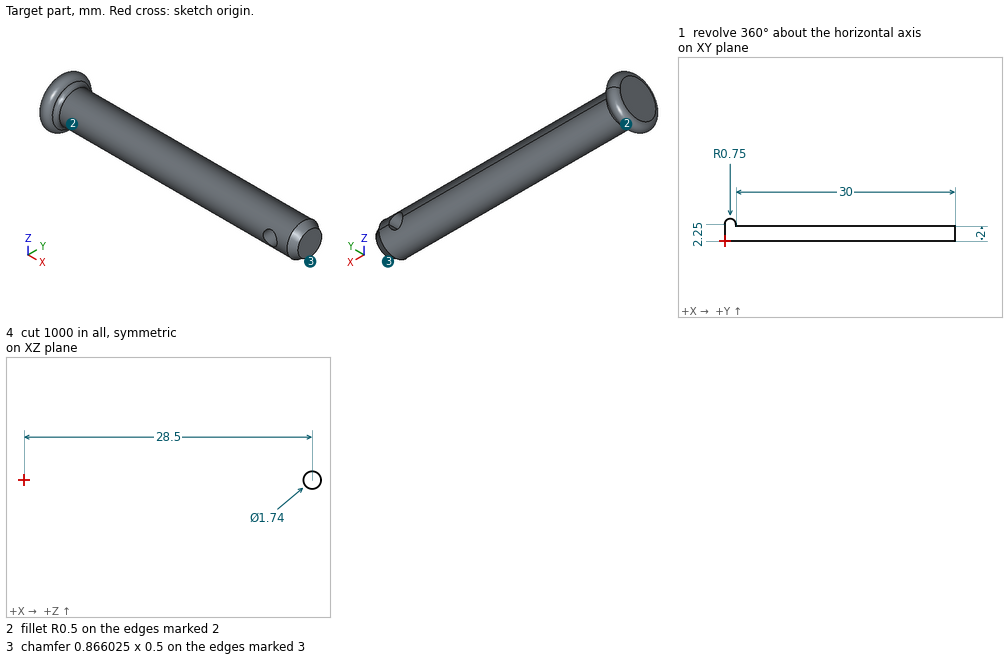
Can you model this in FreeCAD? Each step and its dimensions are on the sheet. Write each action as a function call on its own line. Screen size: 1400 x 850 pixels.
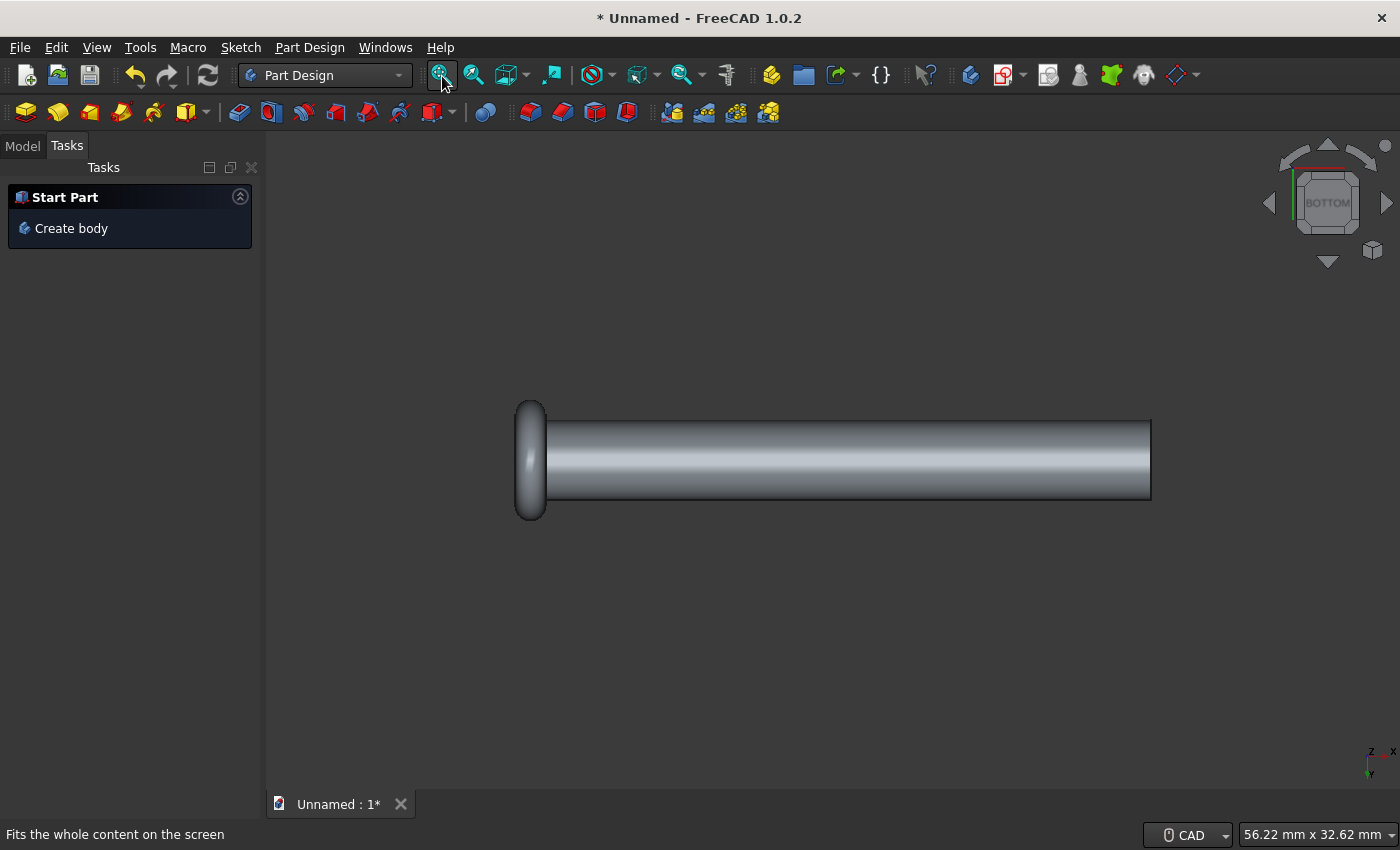
key(4)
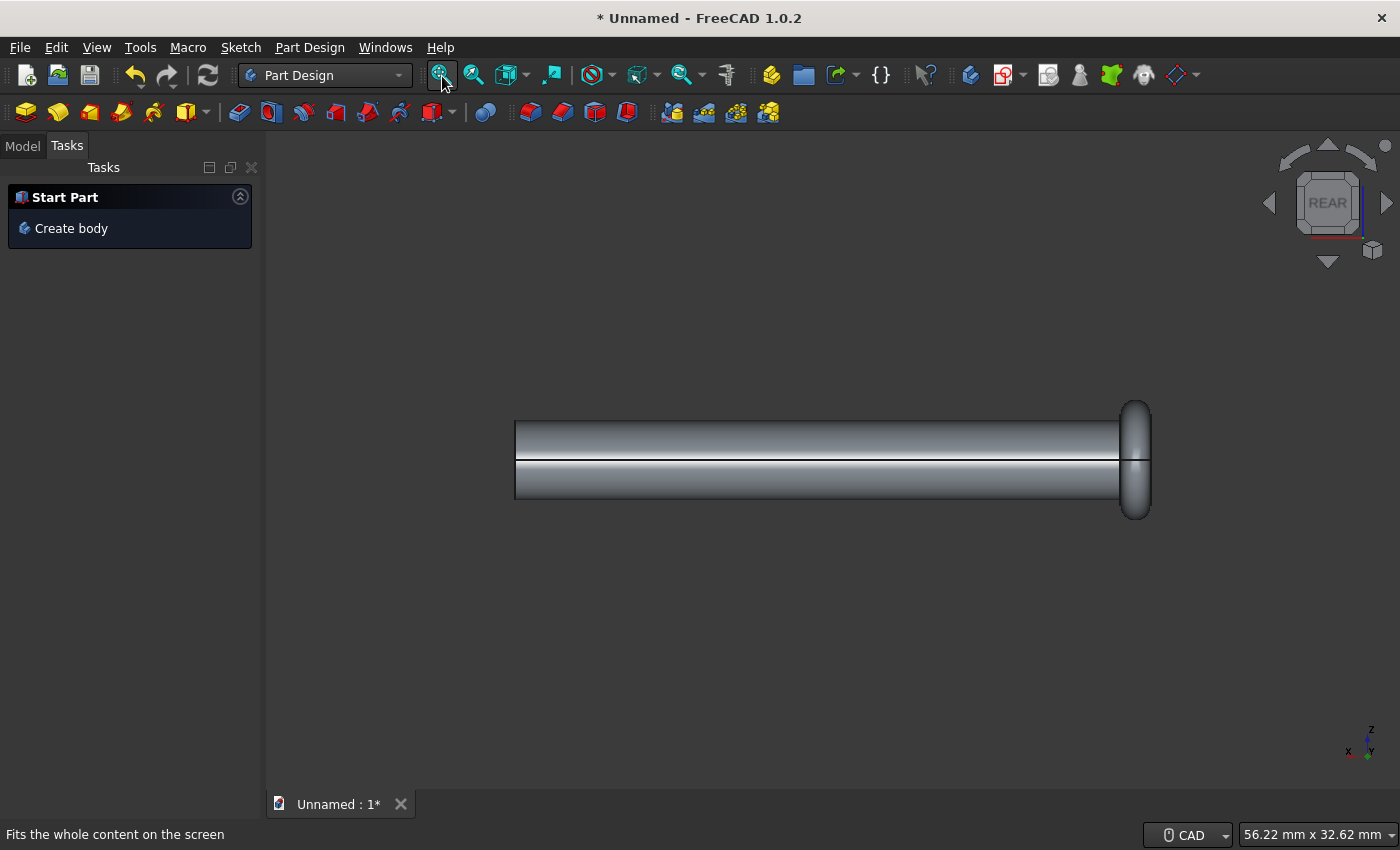
key(6)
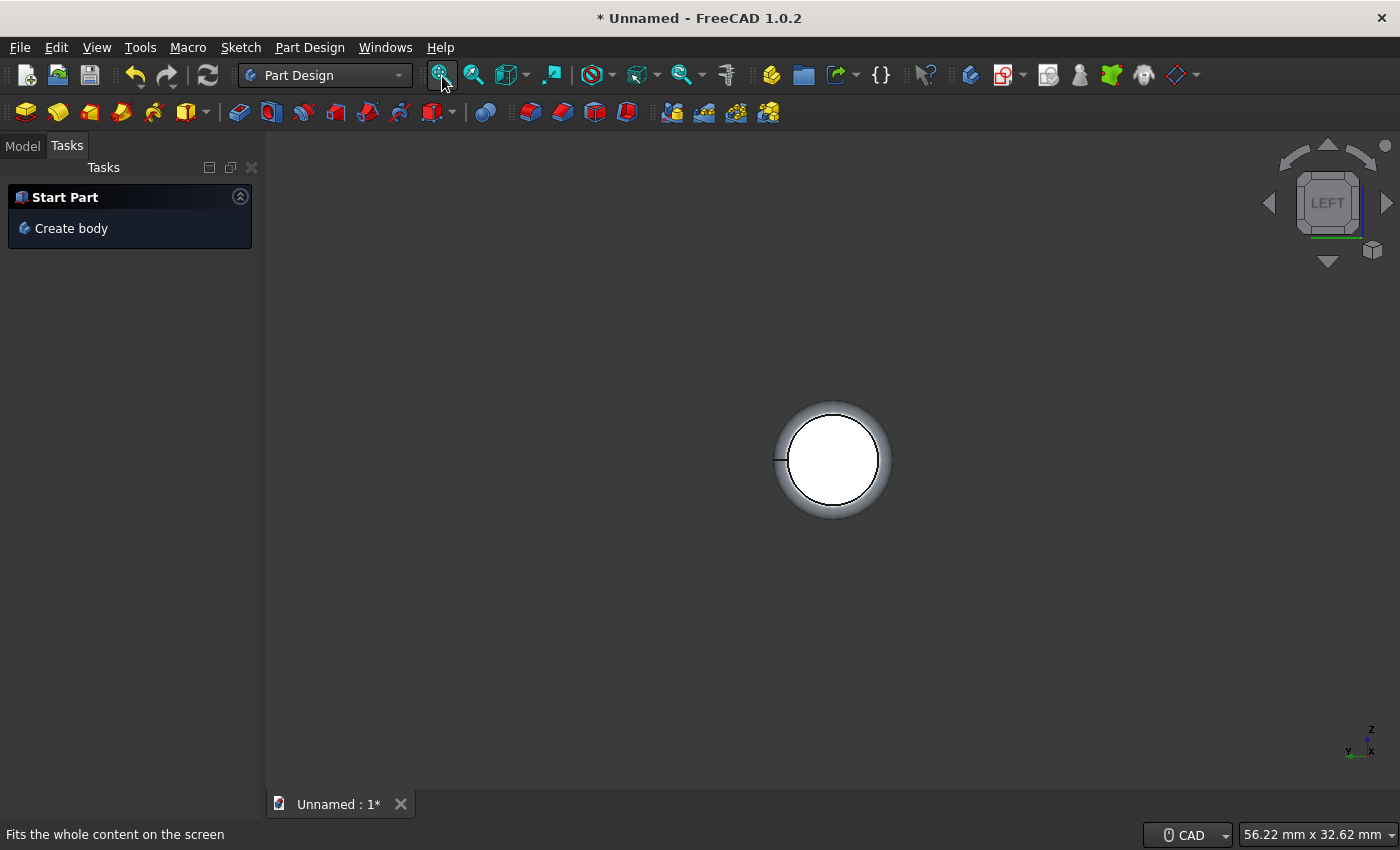
click(442, 76)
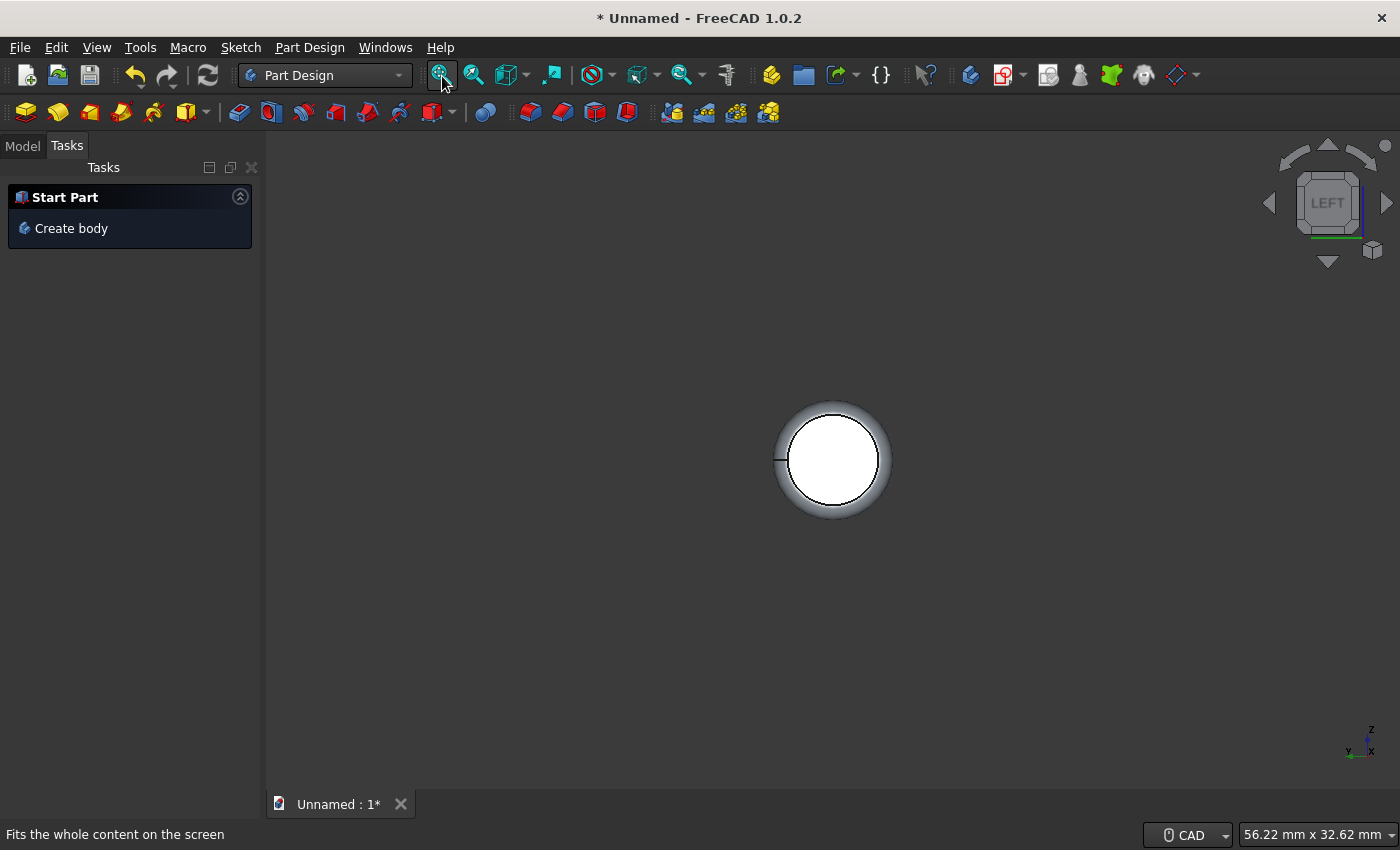
key(v)
key(3)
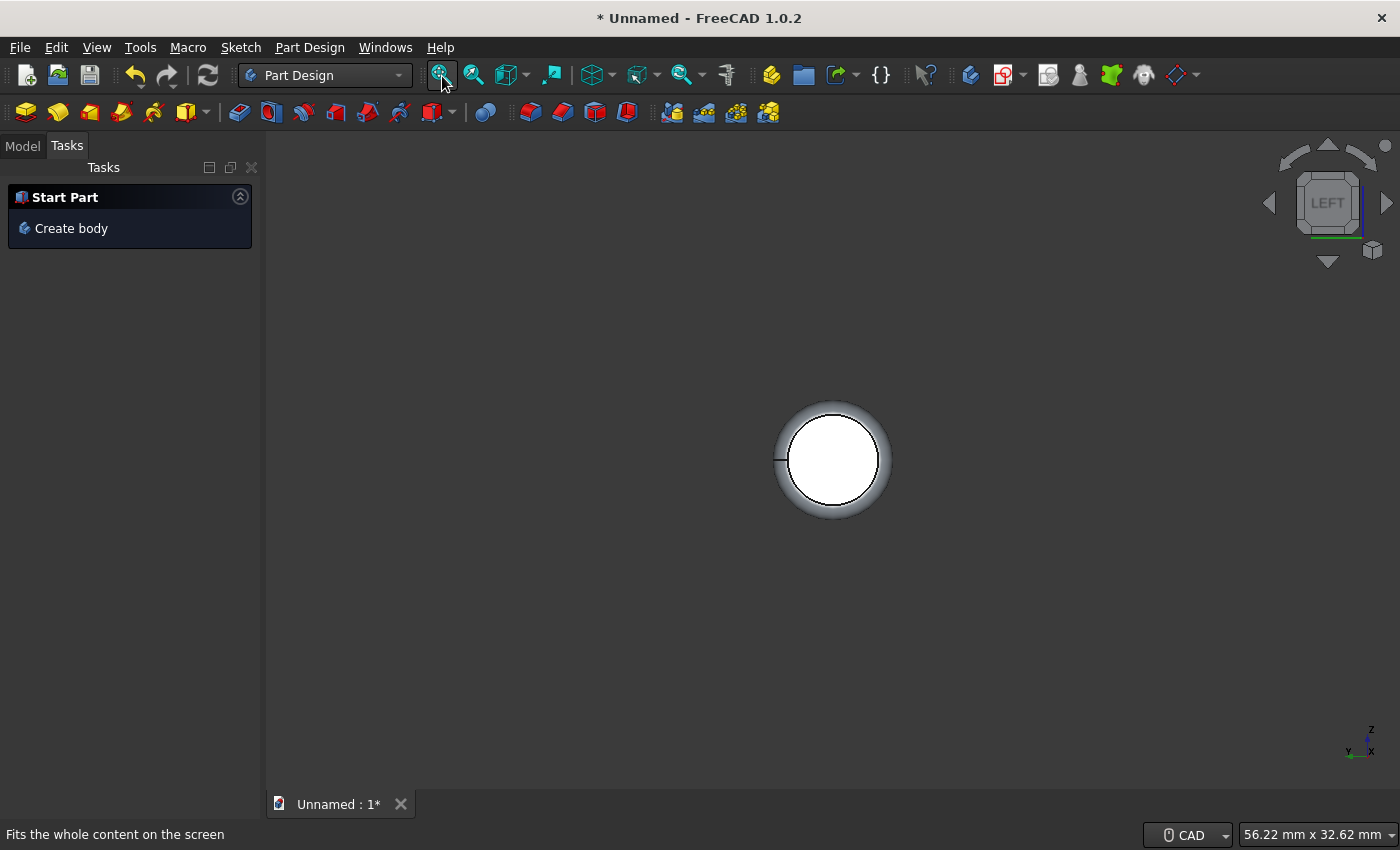
key(0)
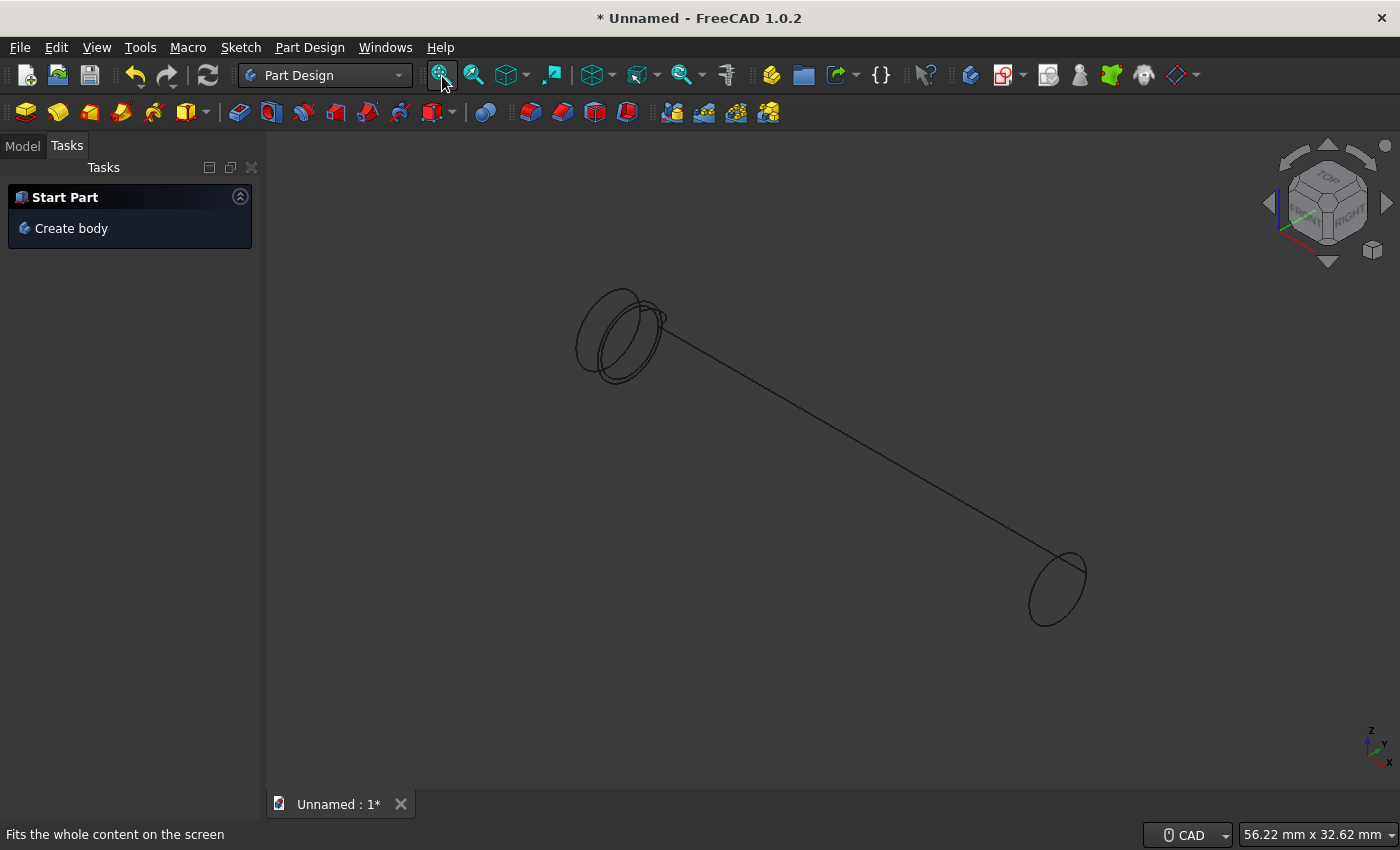
click(621, 378)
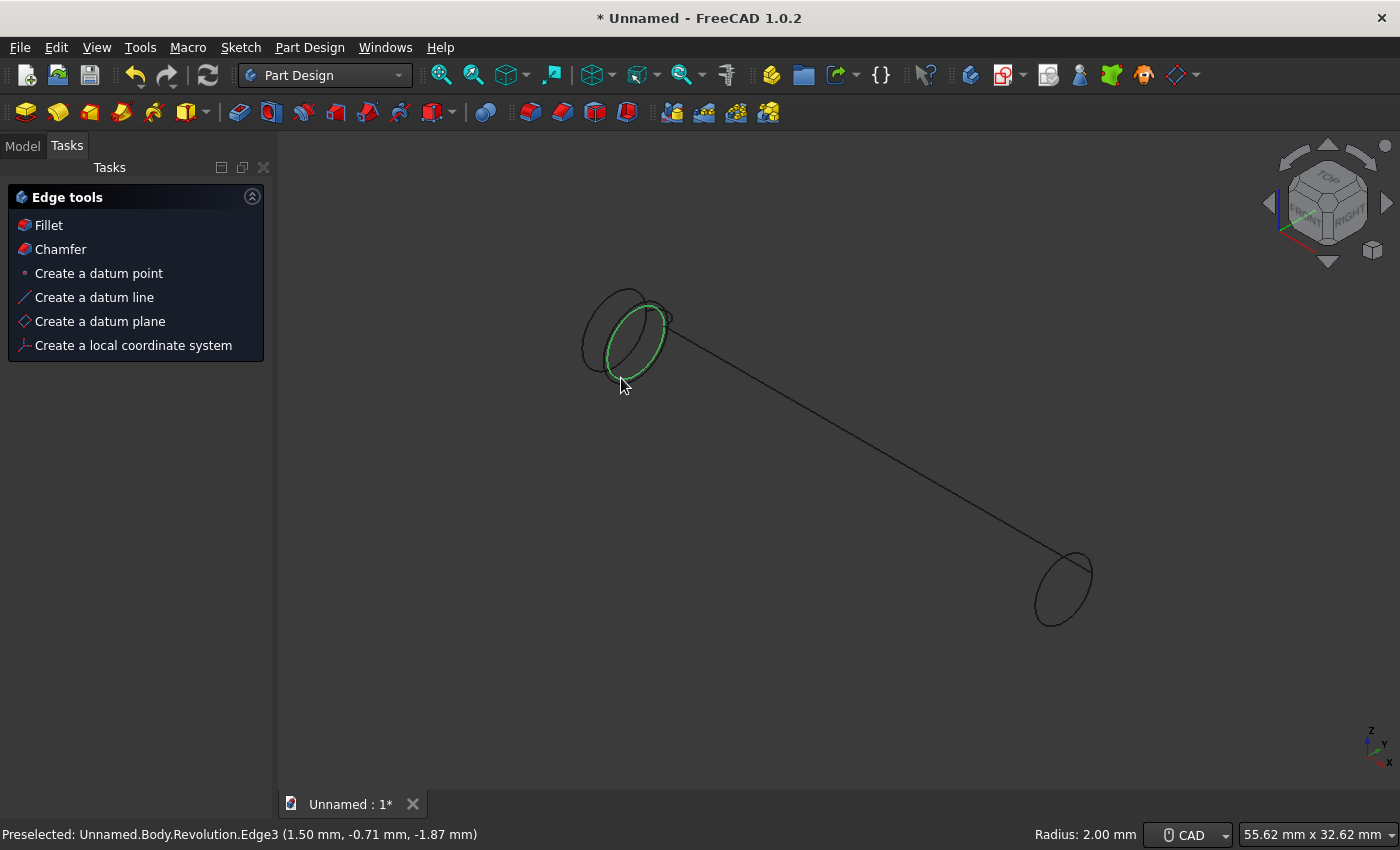
key(v)
key(1)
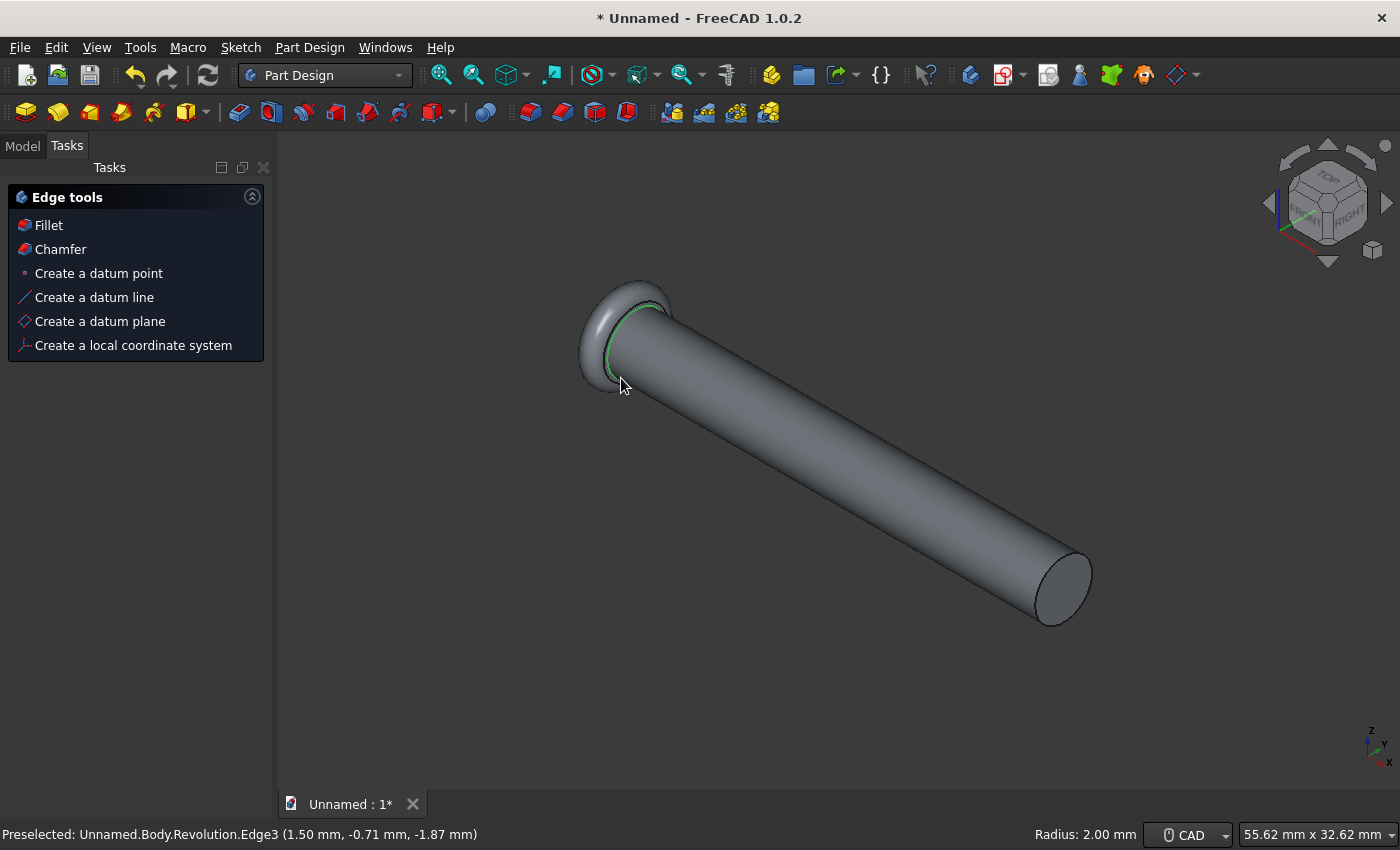
click(532, 112)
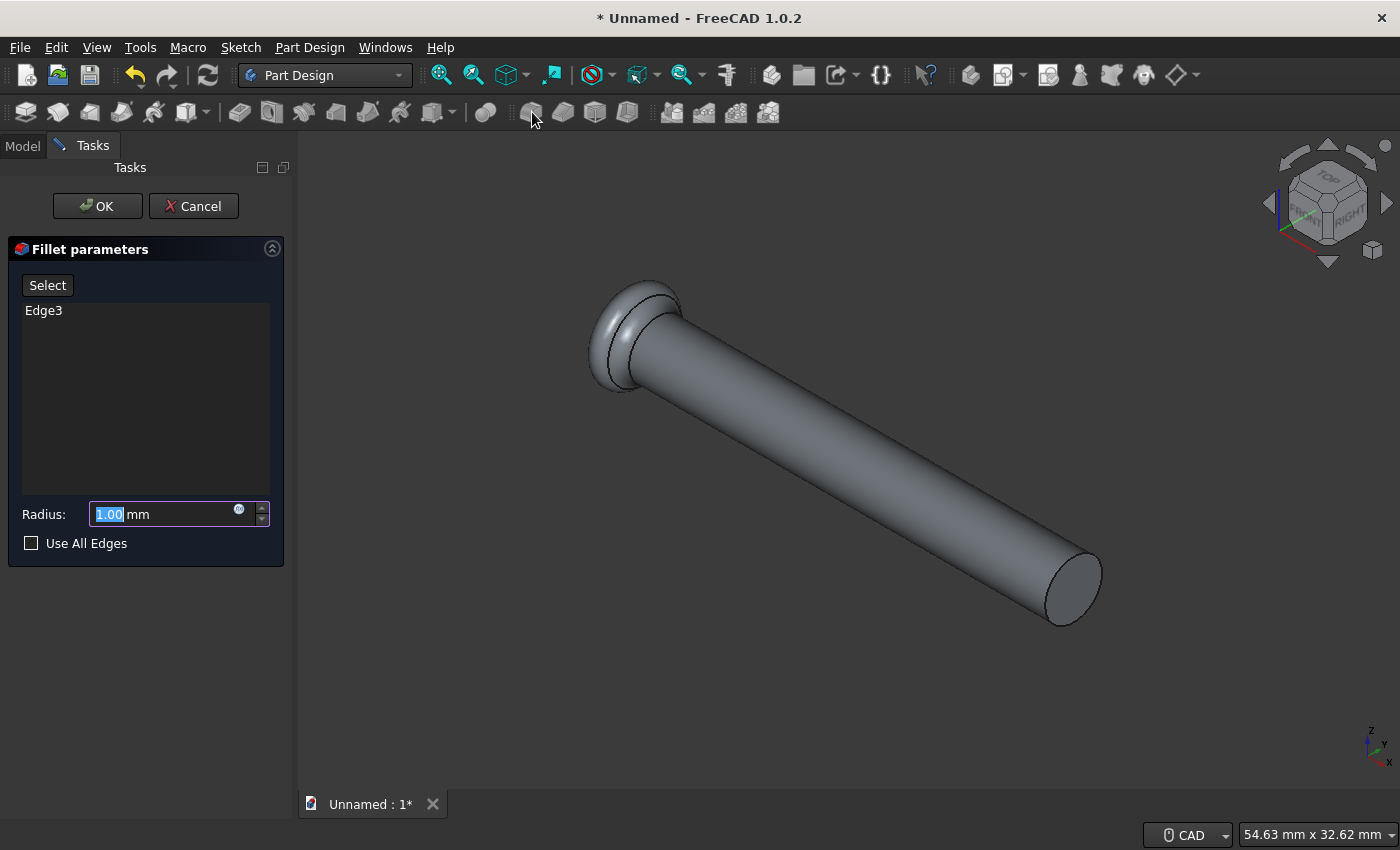
text(0.5)
key(Tab)